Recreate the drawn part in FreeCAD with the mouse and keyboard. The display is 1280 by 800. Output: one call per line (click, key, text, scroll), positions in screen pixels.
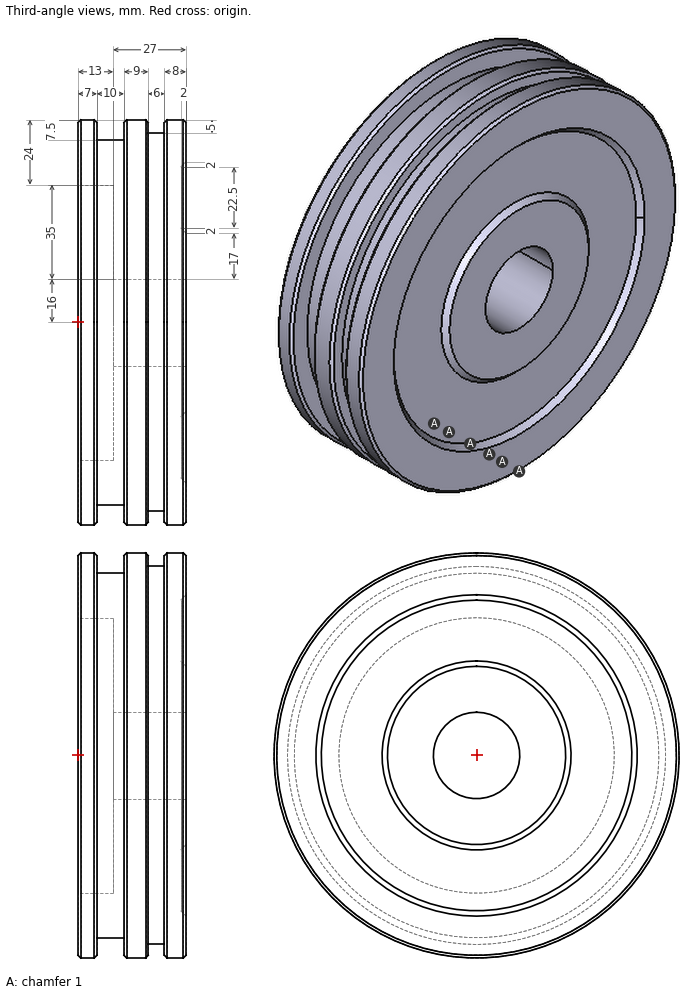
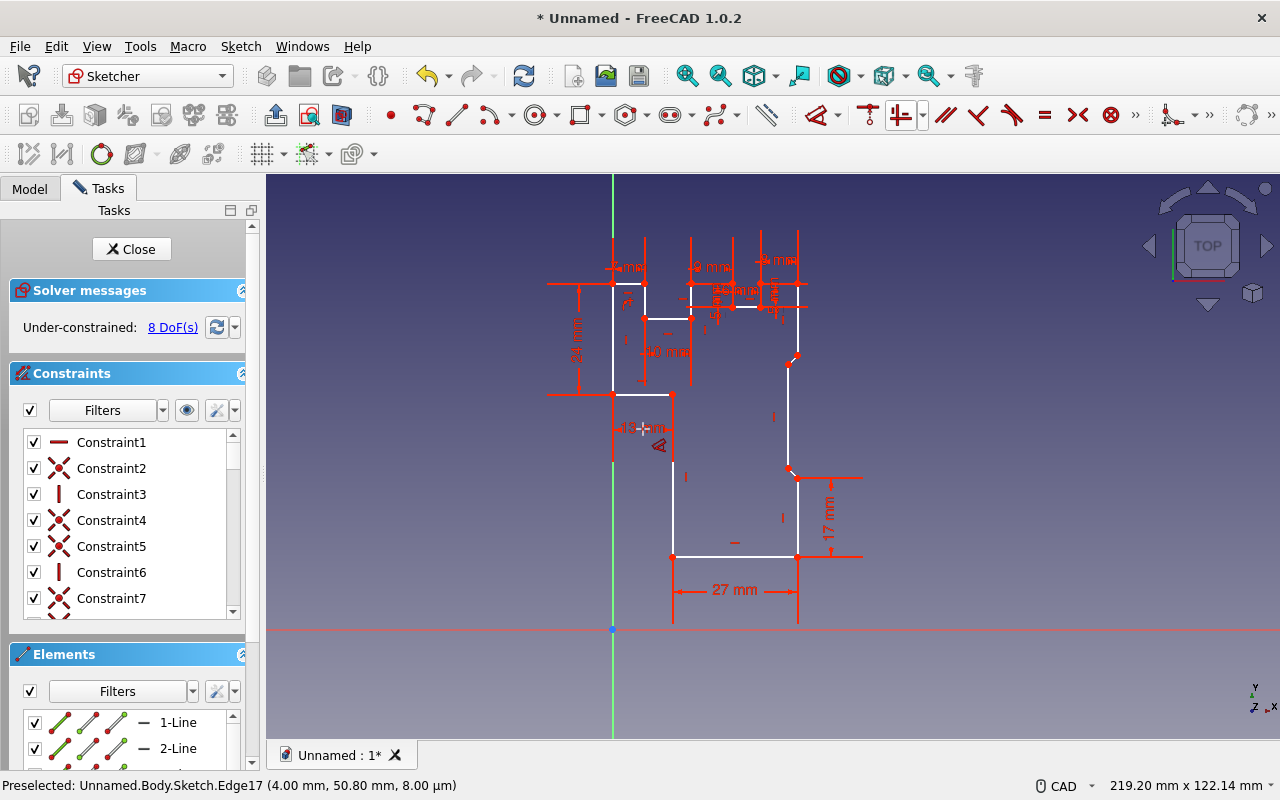
click(673, 444)
click(639, 476)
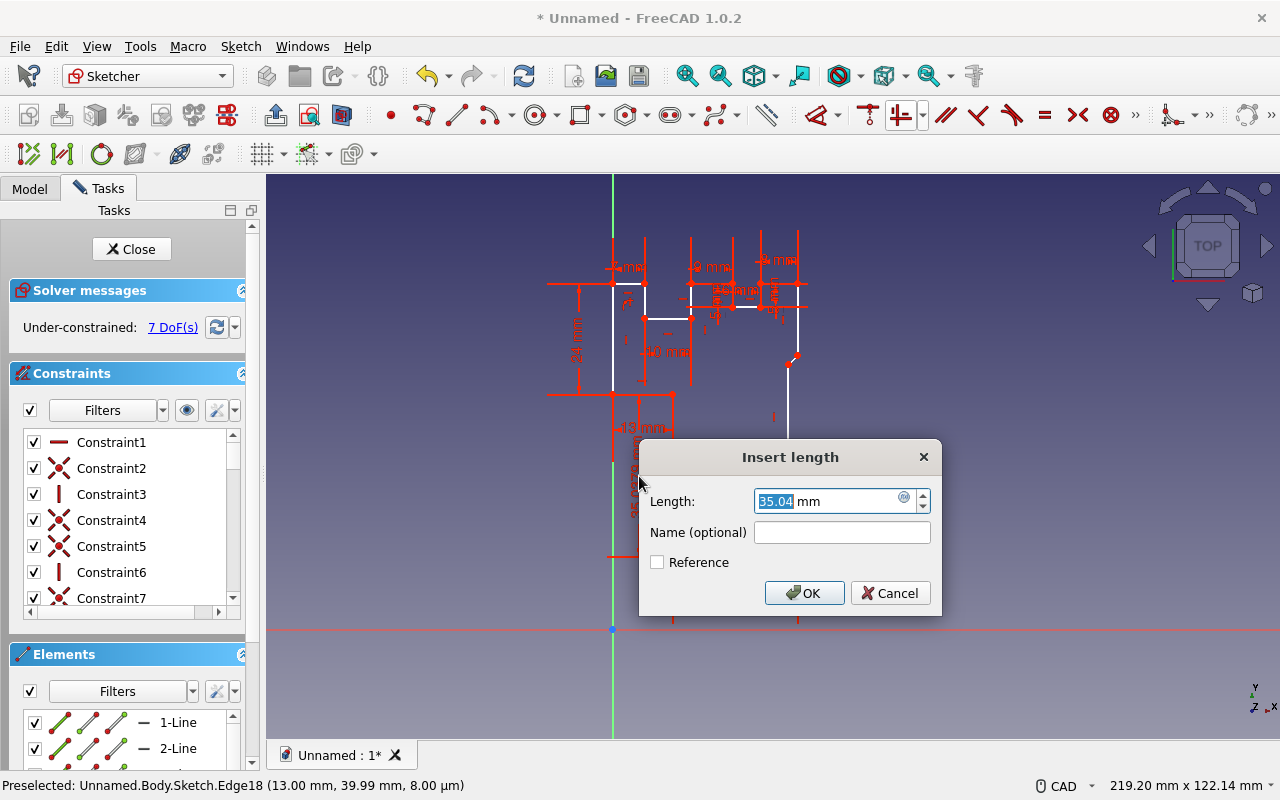
text(35)
key(Return)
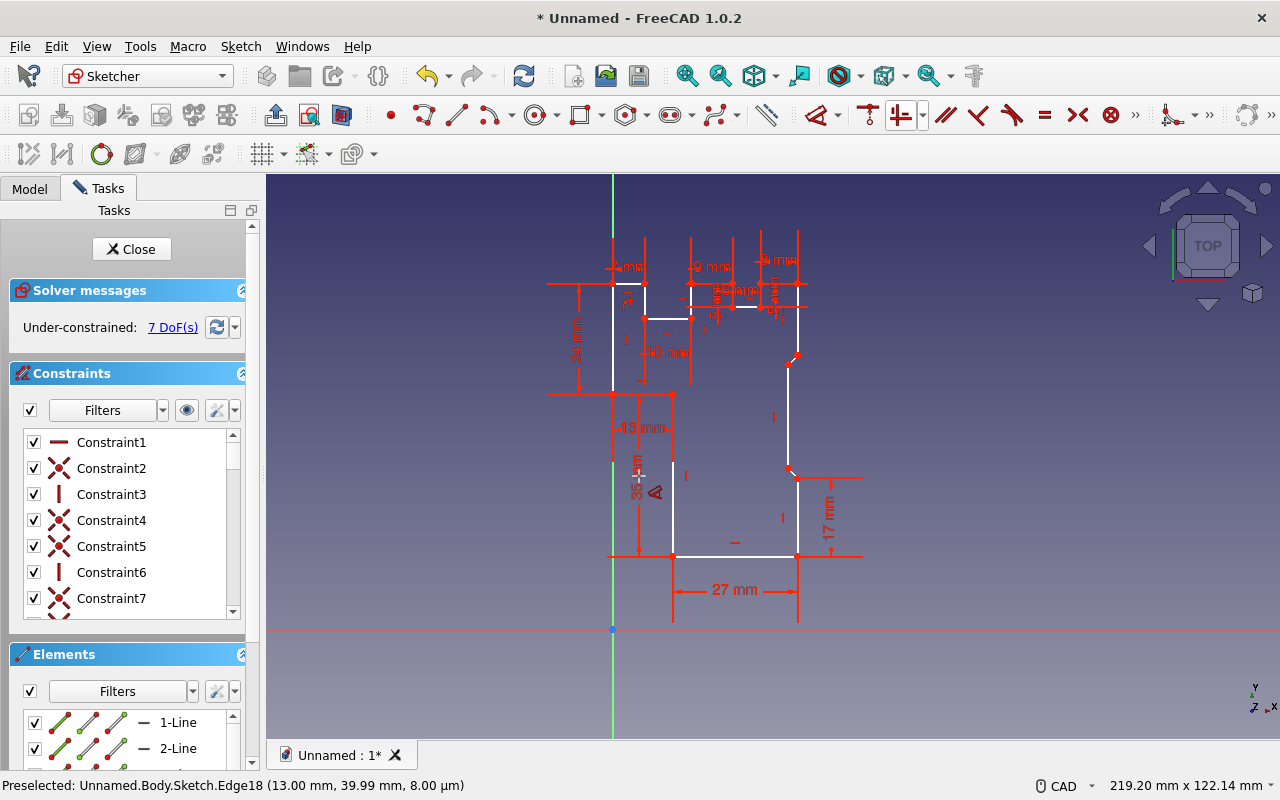
scroll(793, 474, up, 8)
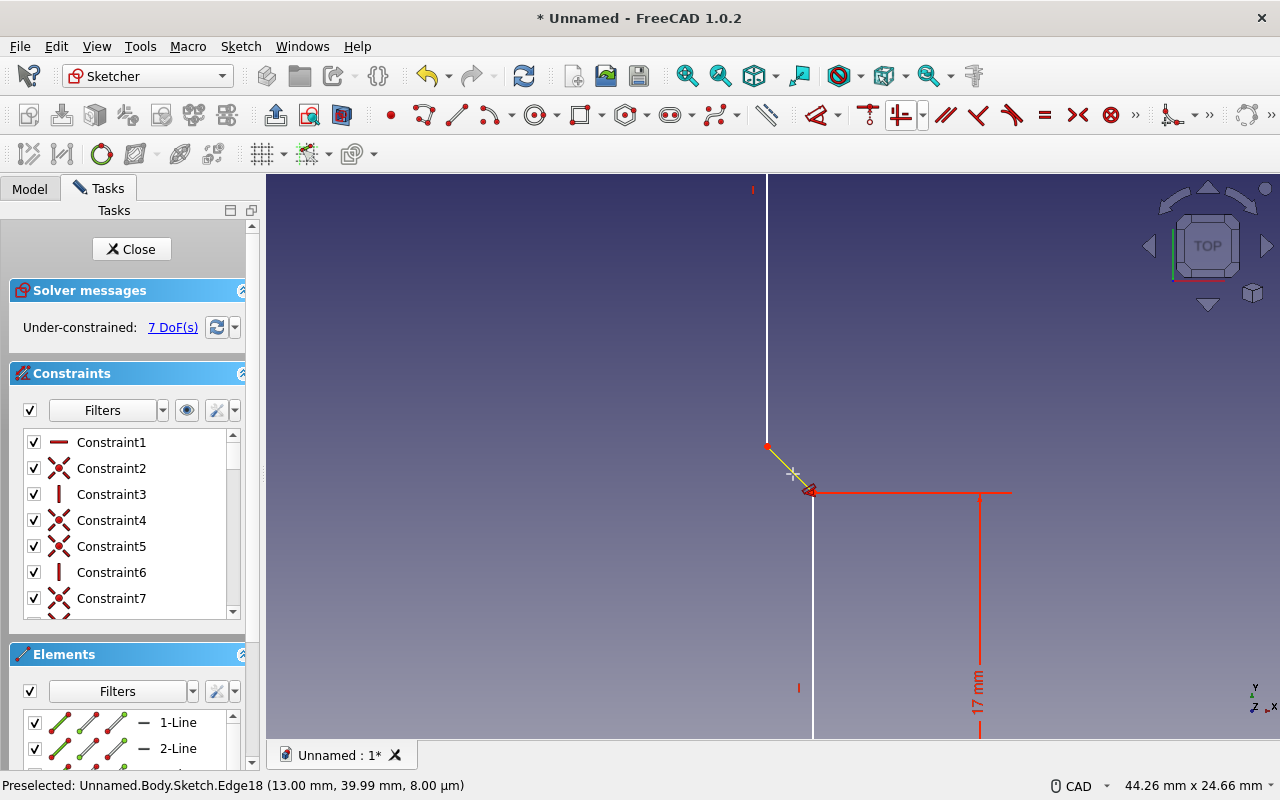
click(790, 470)
click(790, 527)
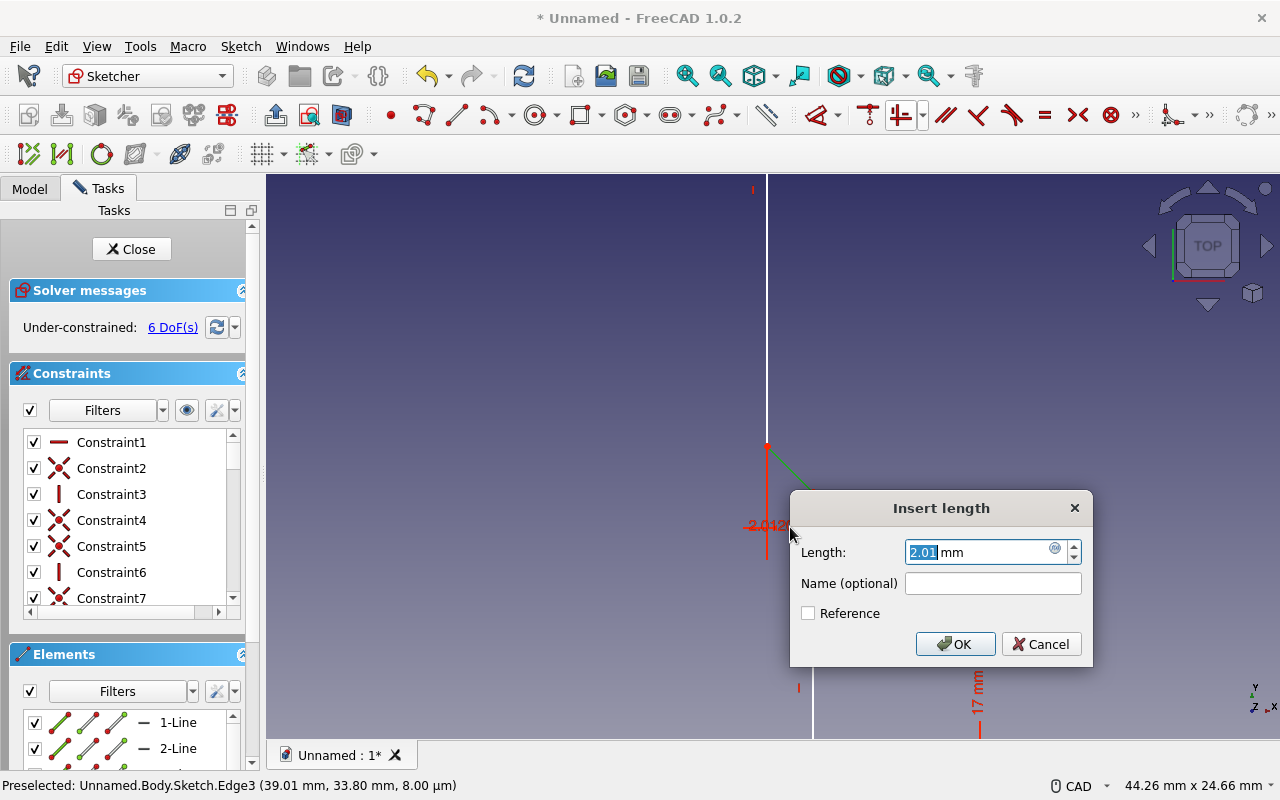
text(2)
key(Return)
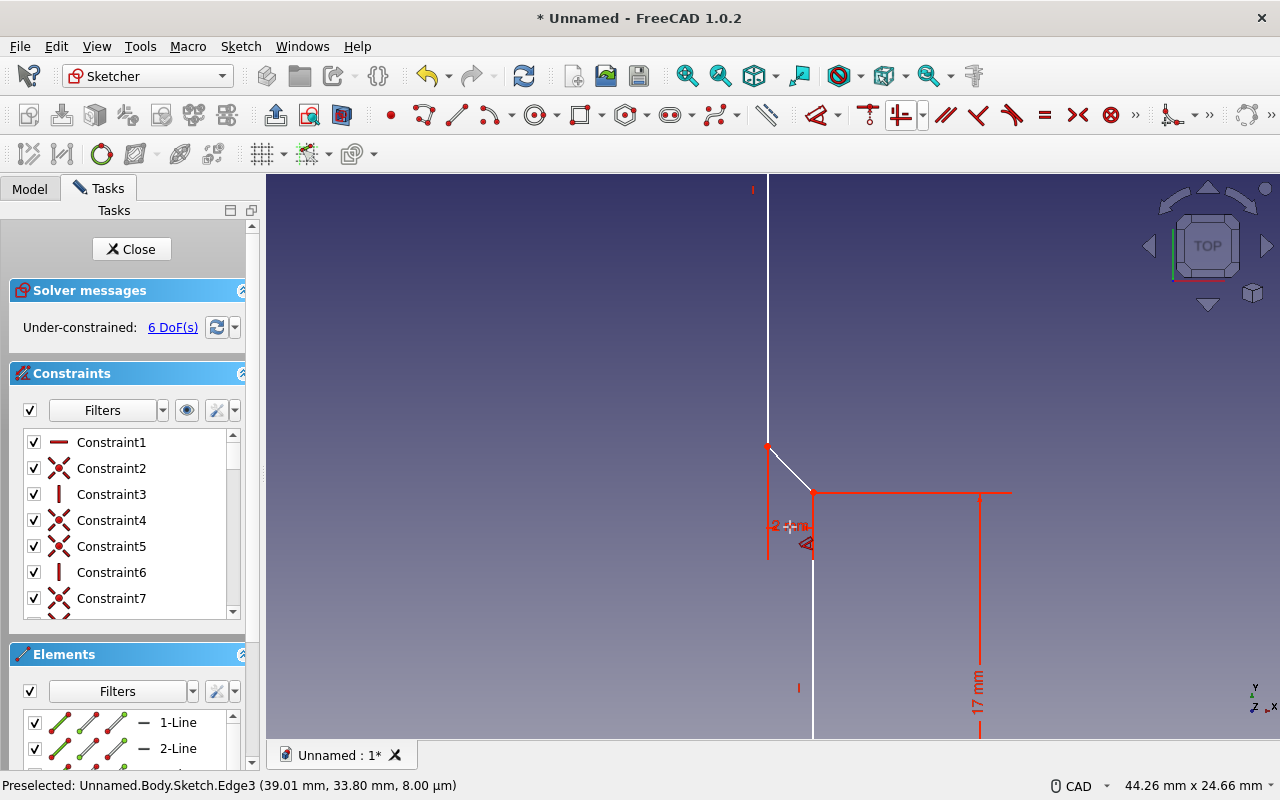
click(800, 479)
click(847, 470)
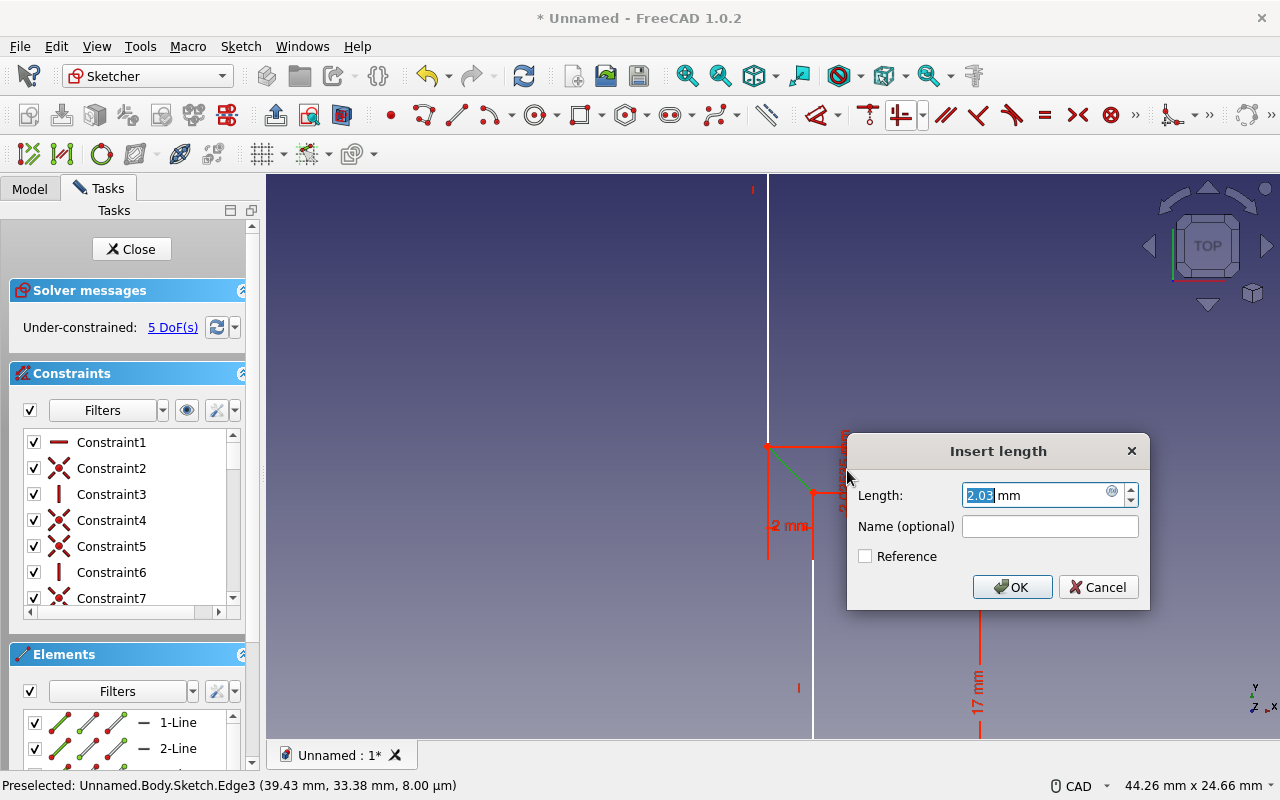
text(2)
key(Return)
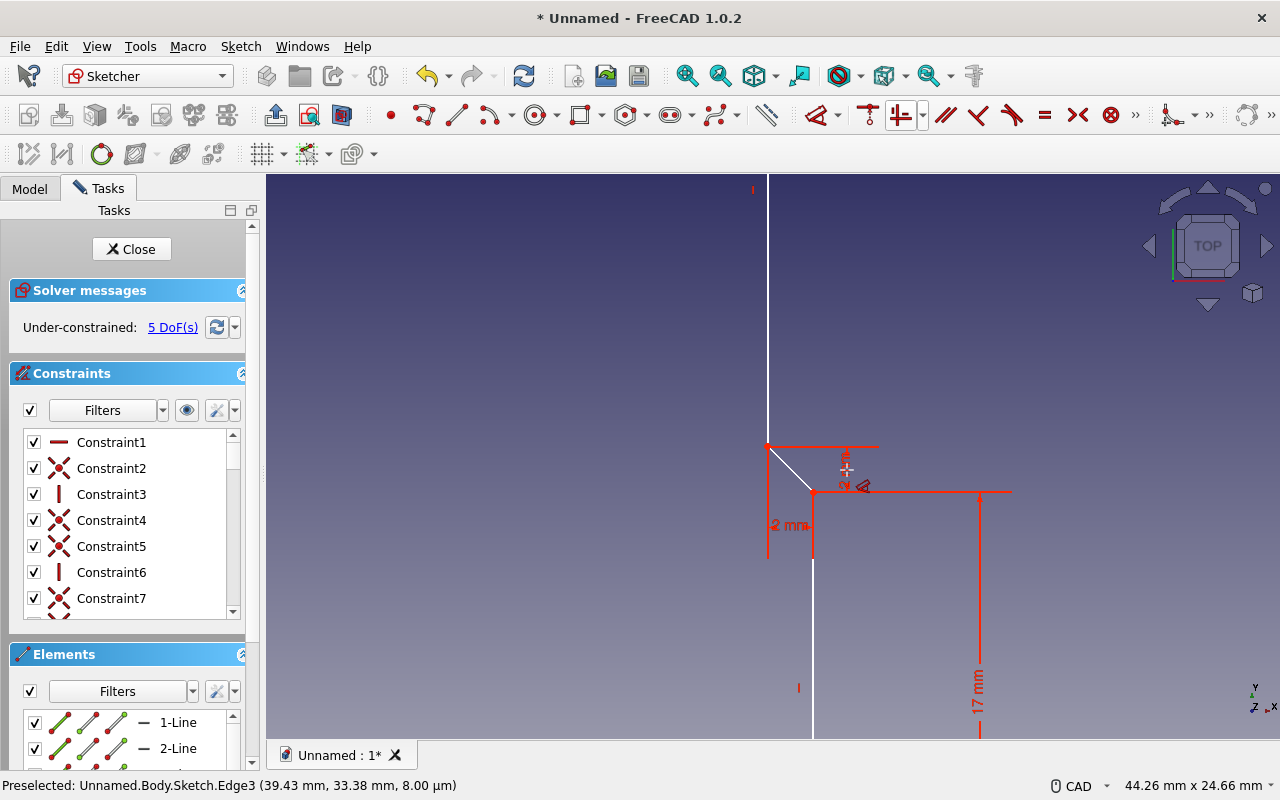
scroll(793, 475, down, 8)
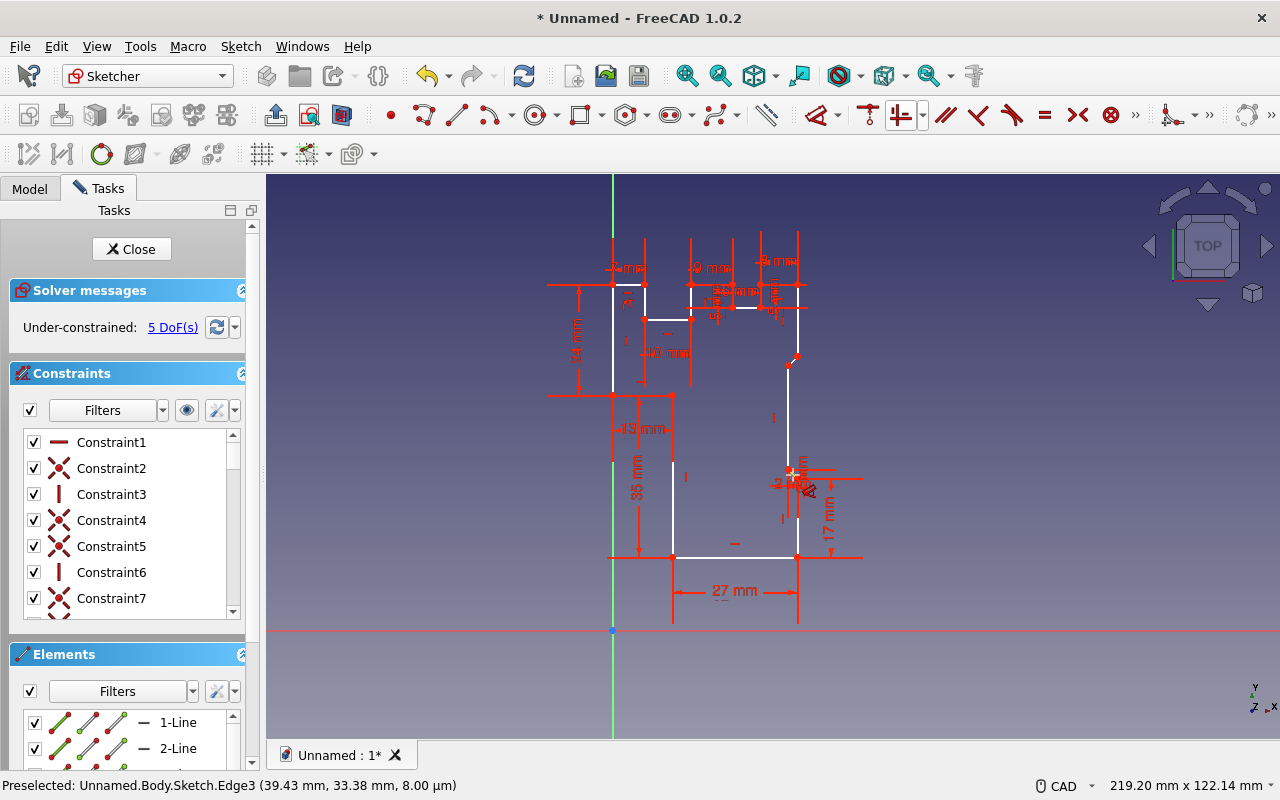
scroll(791, 363, up, 8)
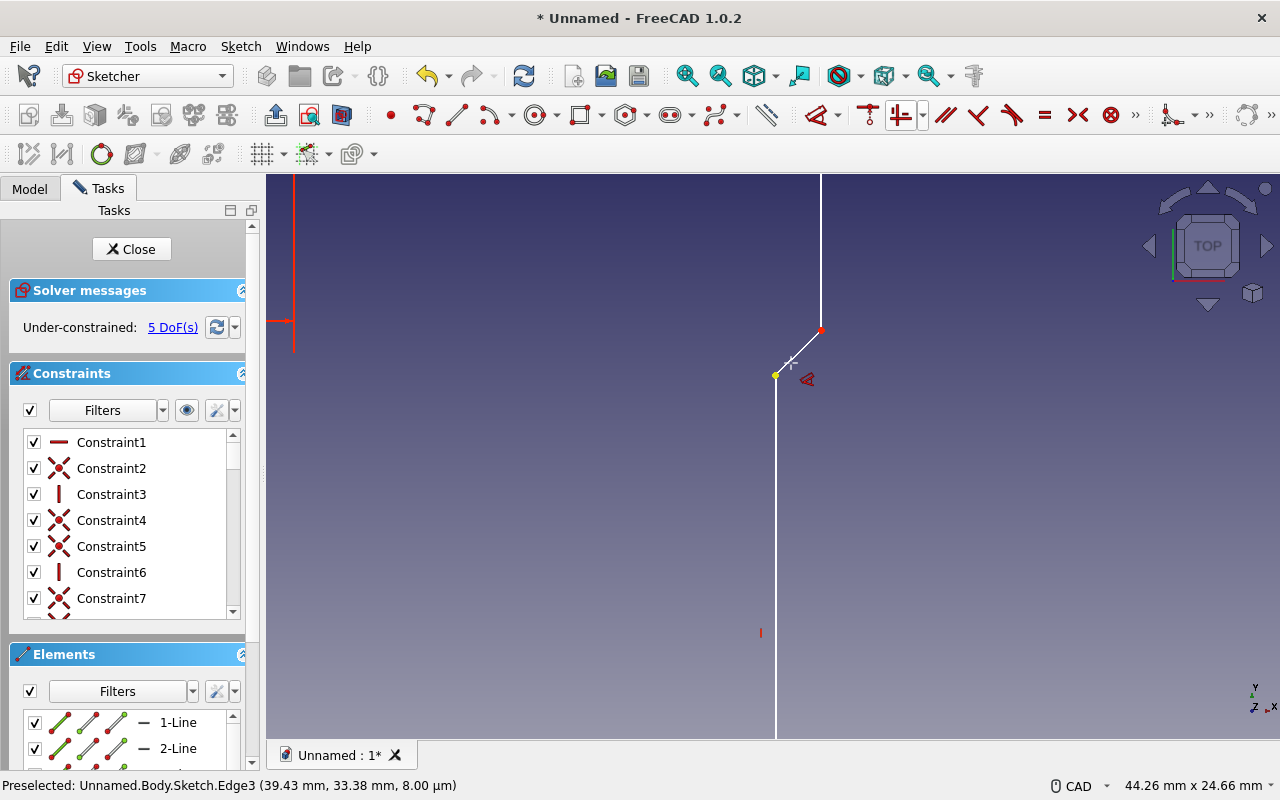
click(789, 362)
click(855, 353)